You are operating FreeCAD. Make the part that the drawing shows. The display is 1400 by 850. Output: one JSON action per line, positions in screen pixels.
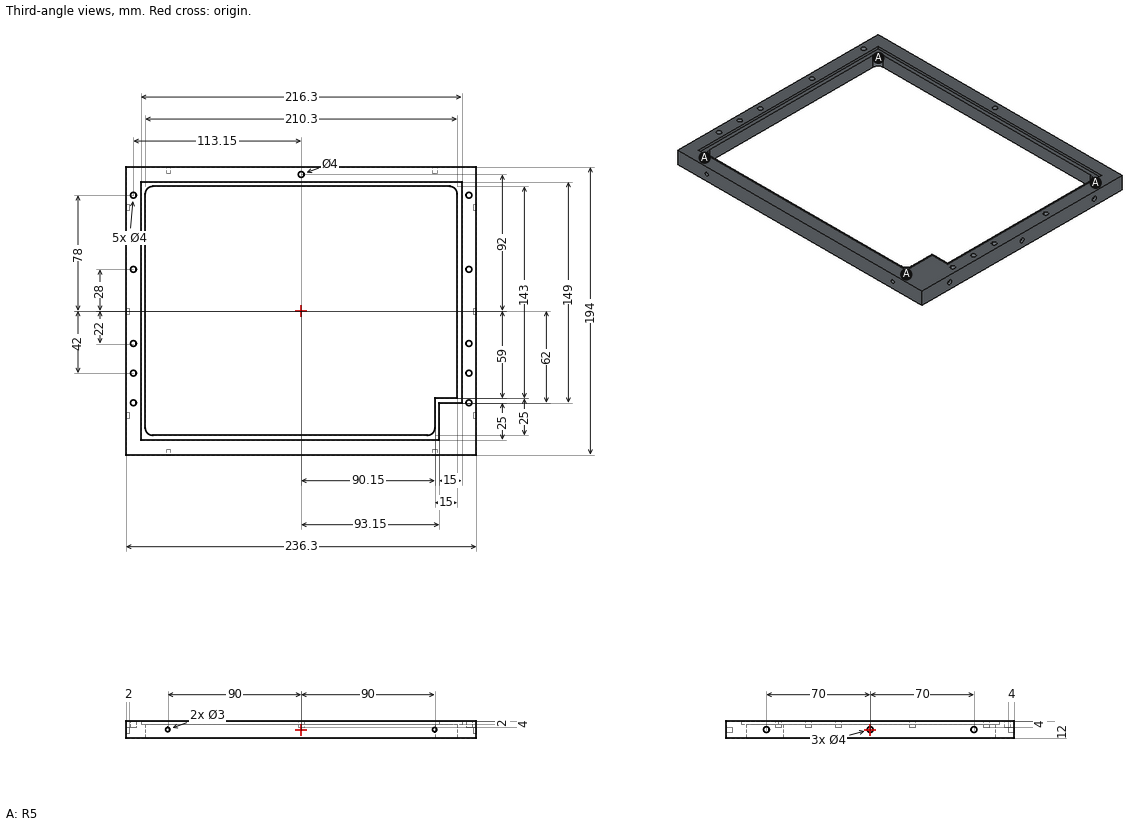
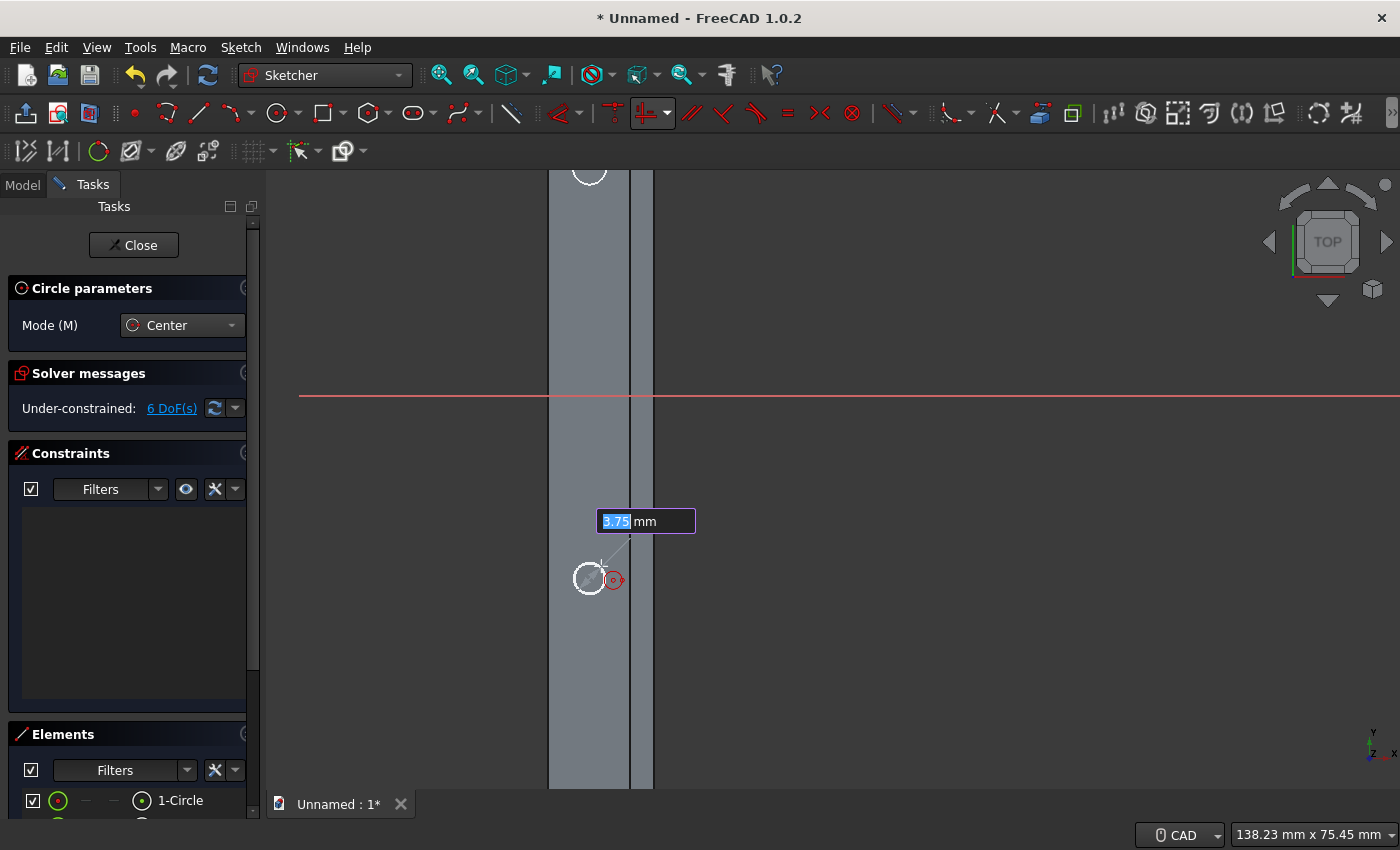
{"action": "left_click", "coordinate": [600, 565]}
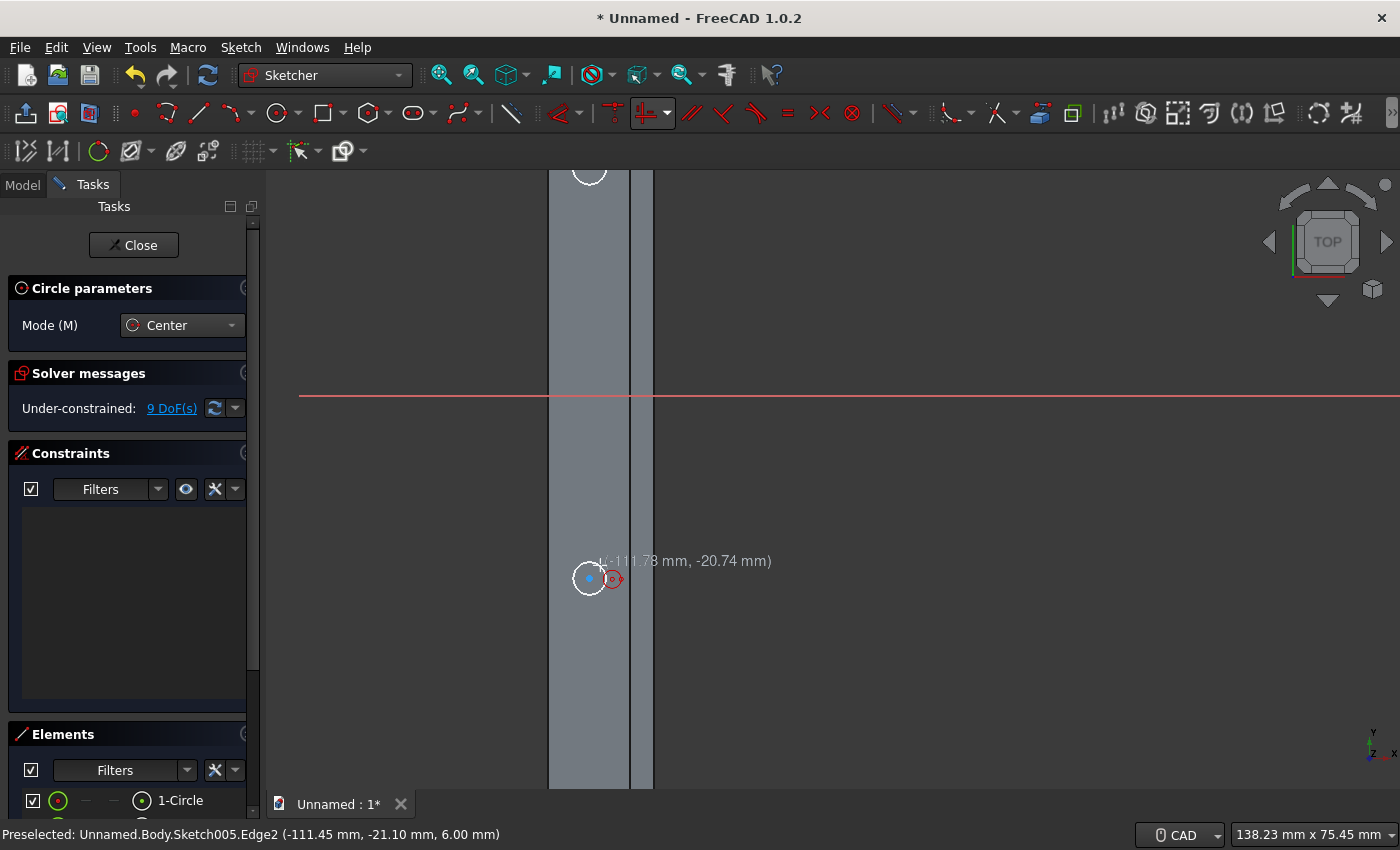
{"action": "scroll", "coordinate": [589, 740], "scroll_direction": "up", "scroll_amount": 2}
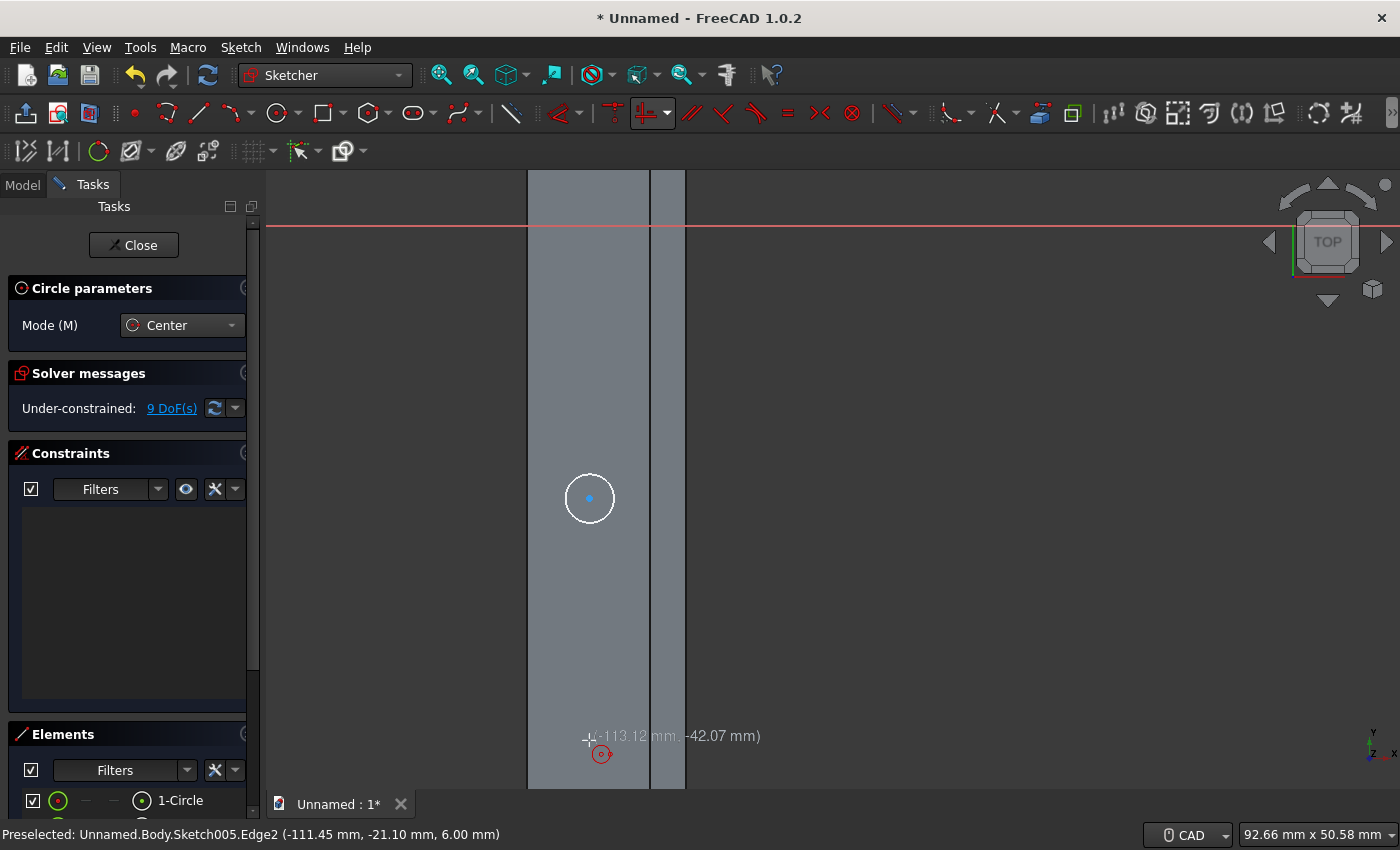
{"action": "scroll", "coordinate": [599, 594], "scroll_direction": "down", "scroll_amount": 7}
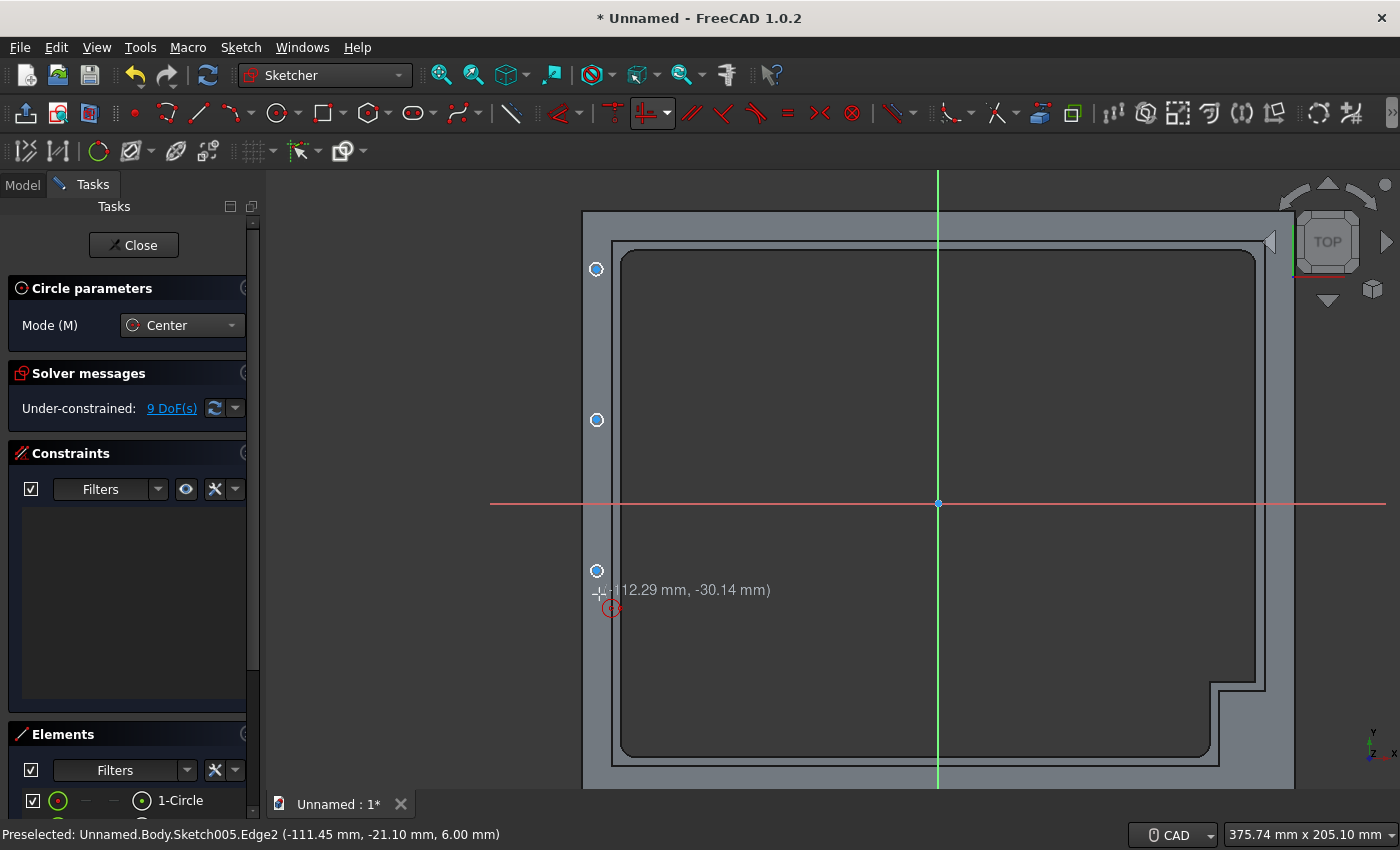
{"action": "left_click", "coordinate": [597, 631]}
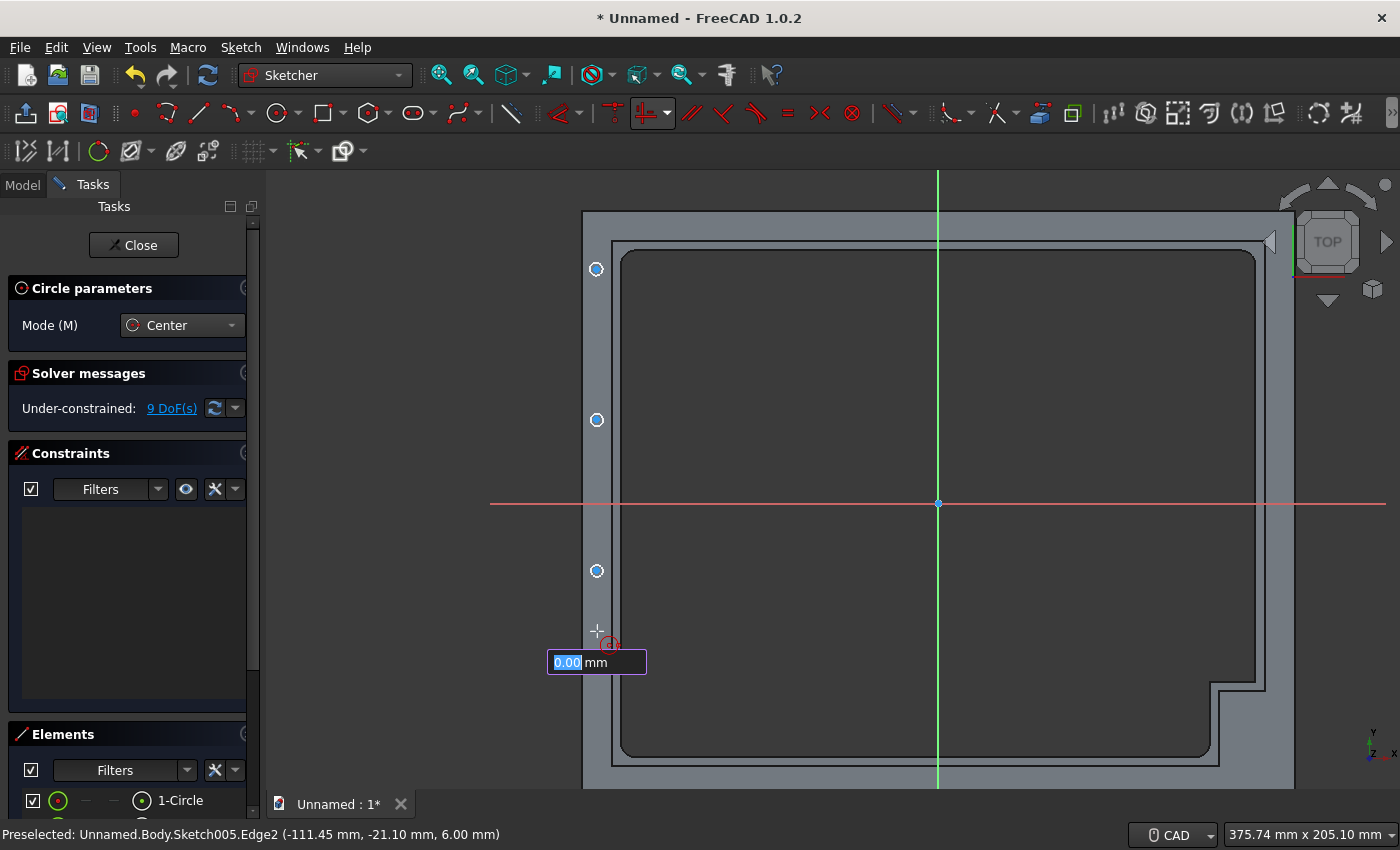
{"action": "scroll", "coordinate": [601, 626], "scroll_direction": "up", "scroll_amount": 5}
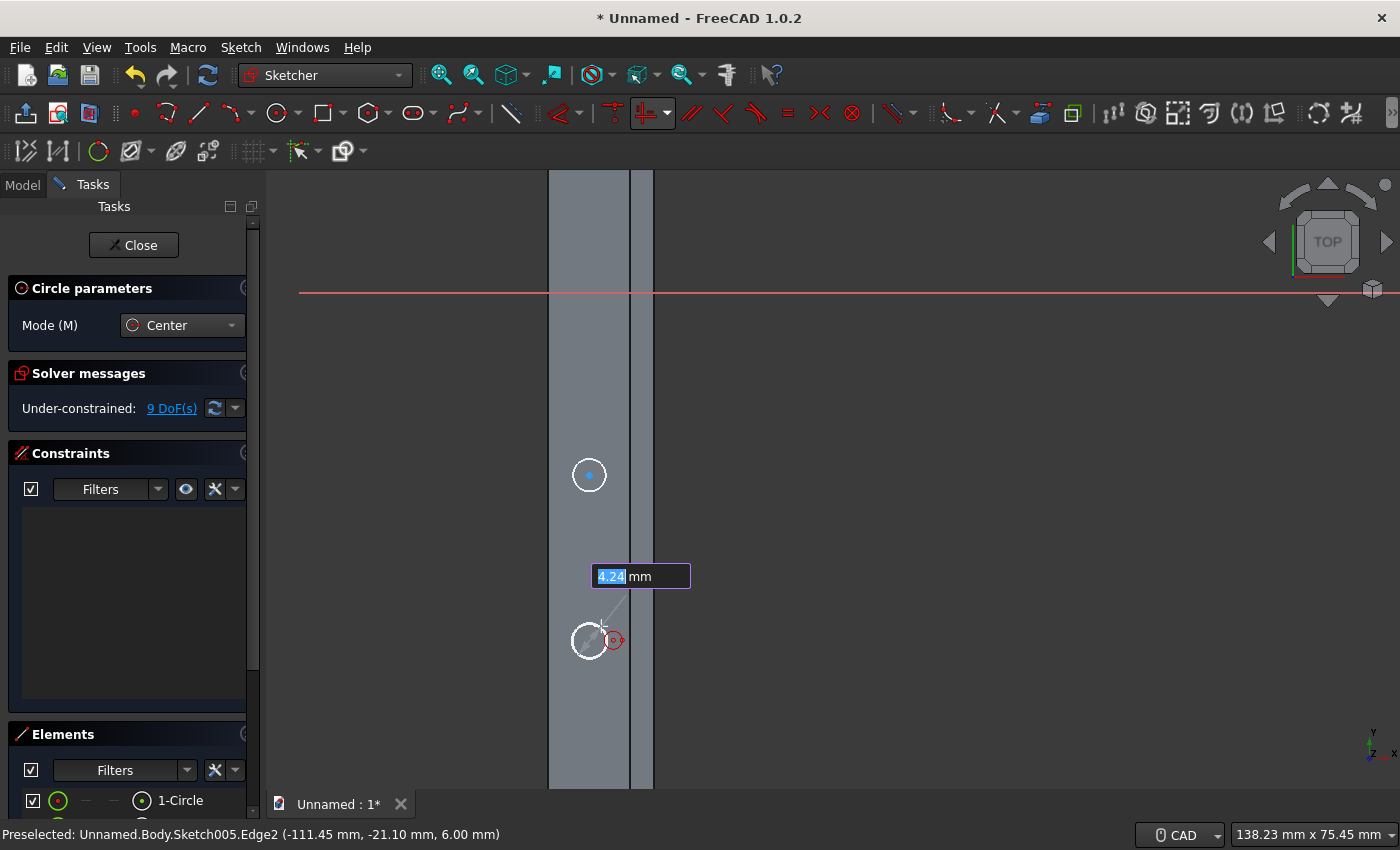
{"action": "left_click", "coordinate": [600, 626]}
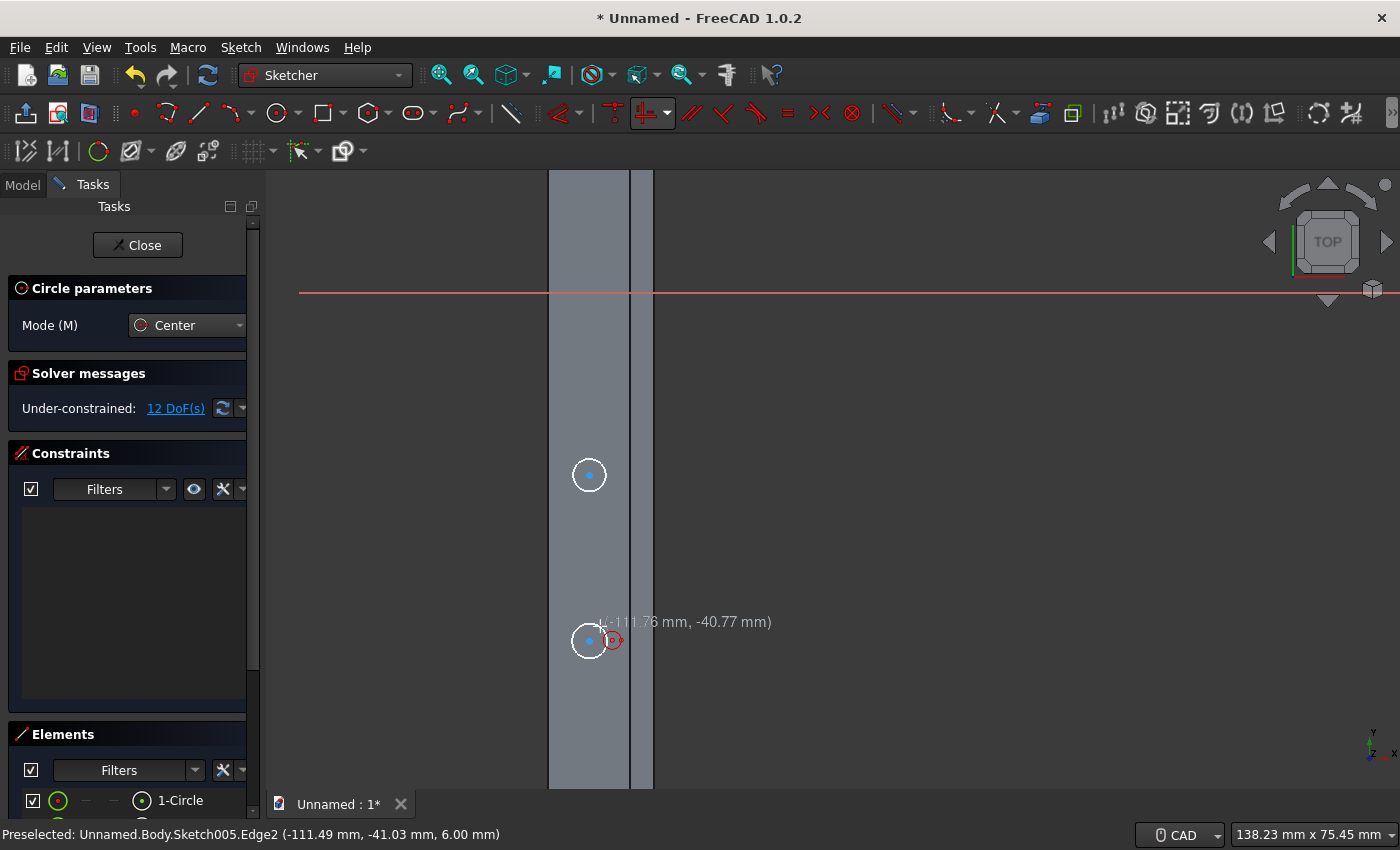
{"action": "scroll", "coordinate": [602, 626], "scroll_direction": "down", "scroll_amount": 5}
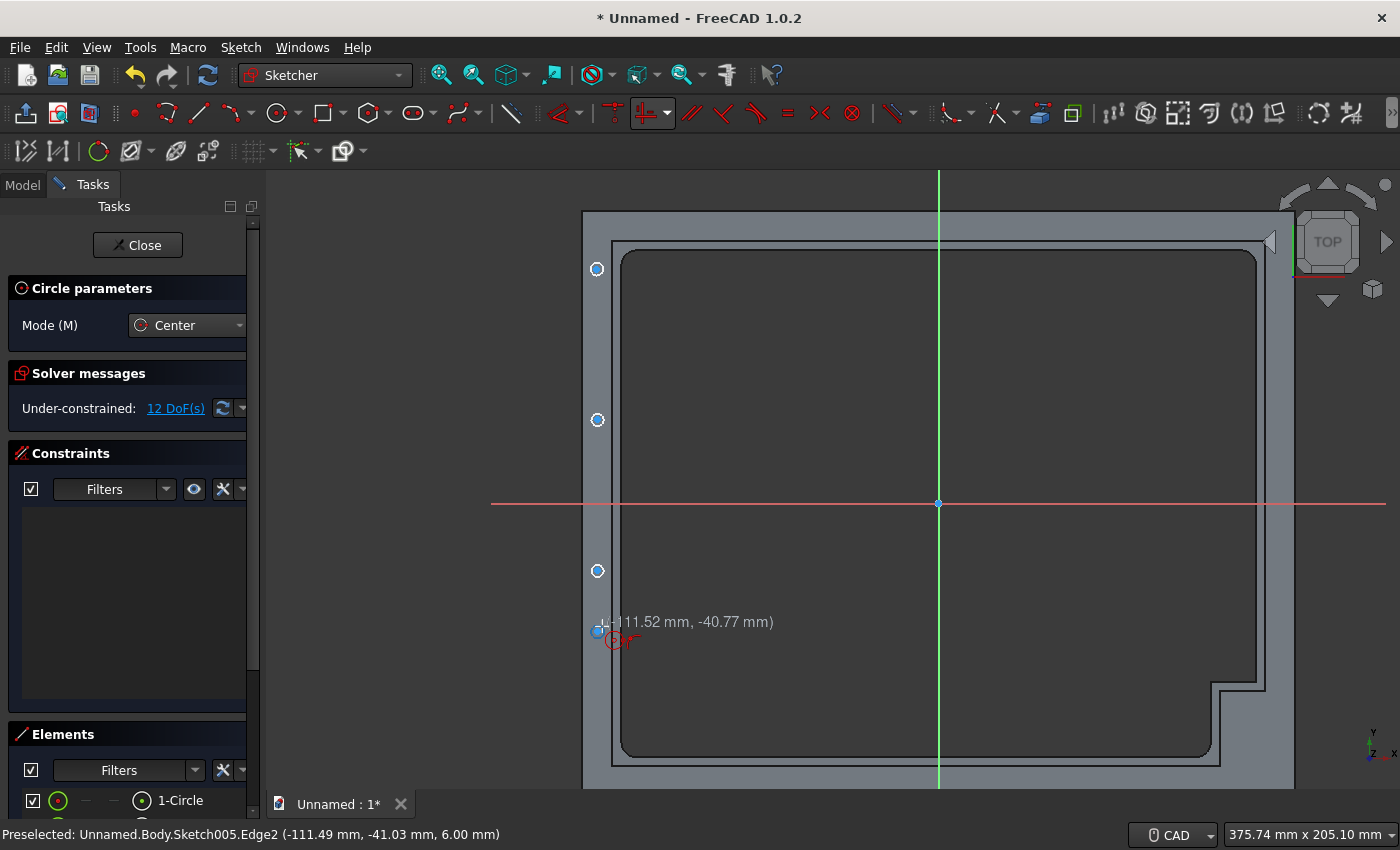
{"action": "scroll", "coordinate": [597, 691], "scroll_direction": "up", "scroll_amount": 7}